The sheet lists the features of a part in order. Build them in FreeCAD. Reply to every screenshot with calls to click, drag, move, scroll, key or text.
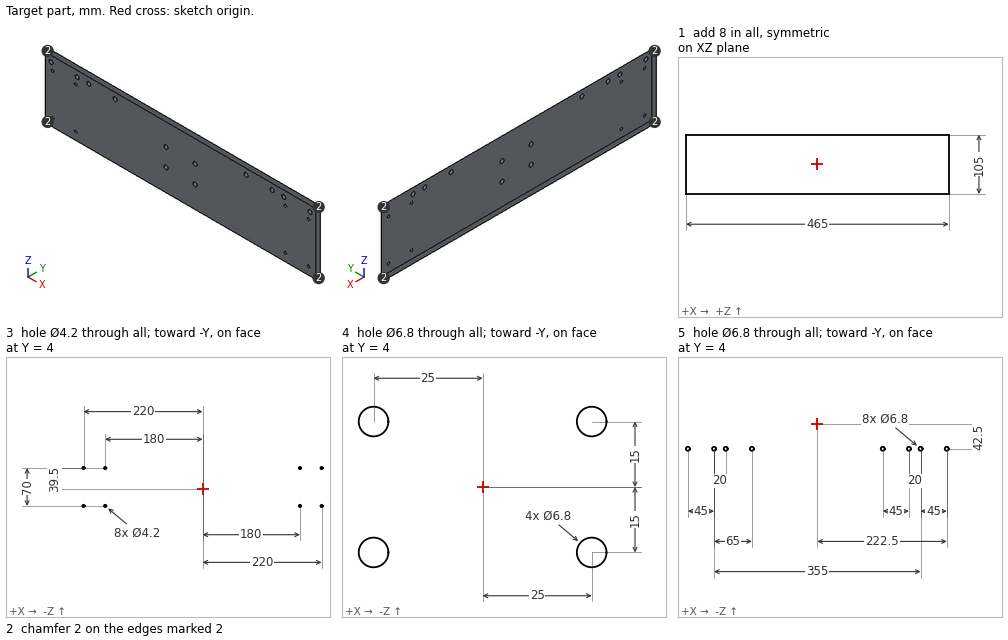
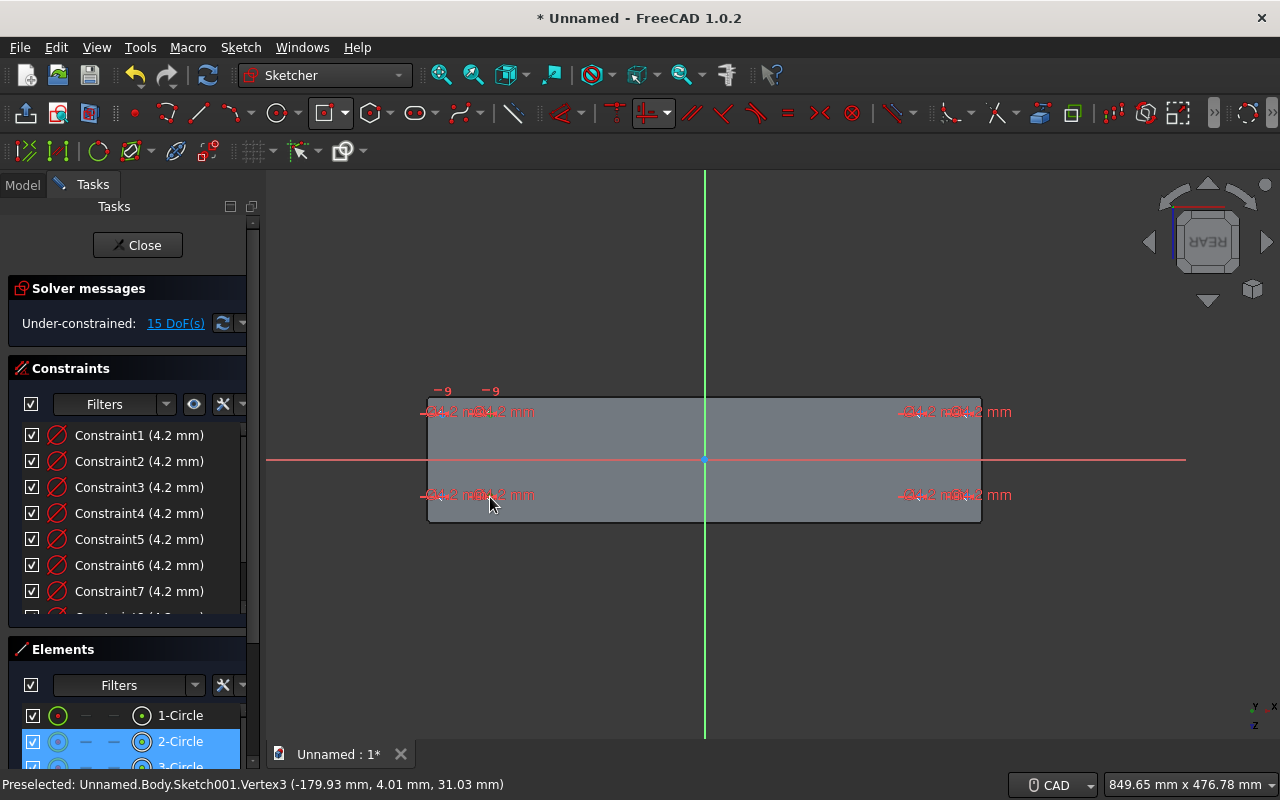
click(670, 114)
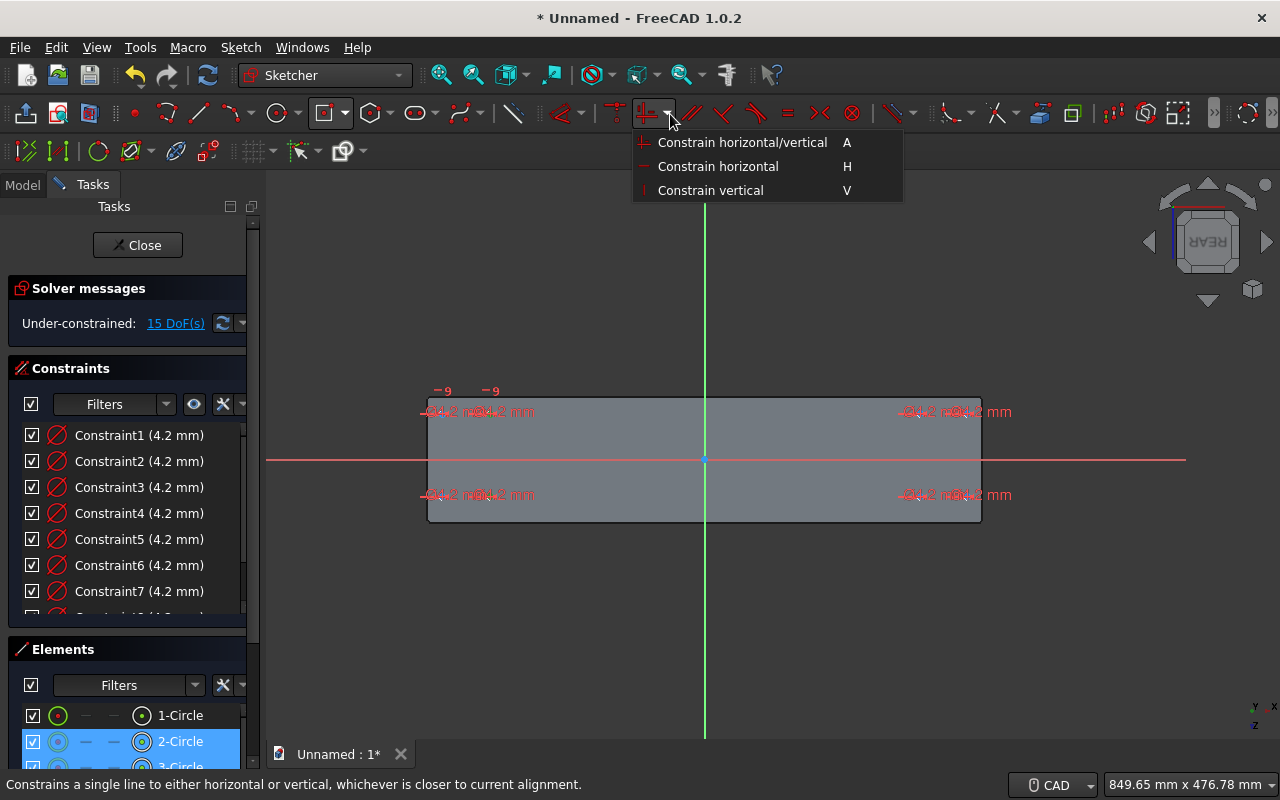
click(768, 190)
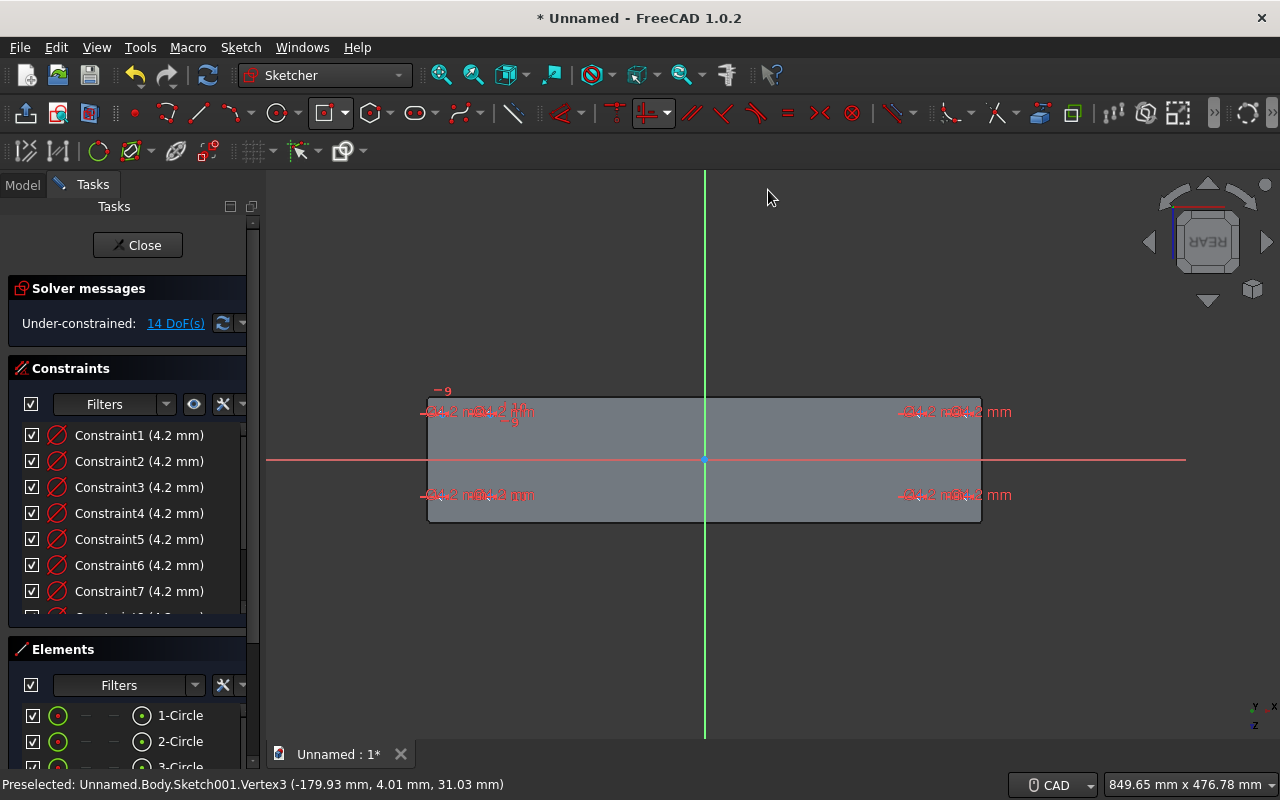
click(442, 414)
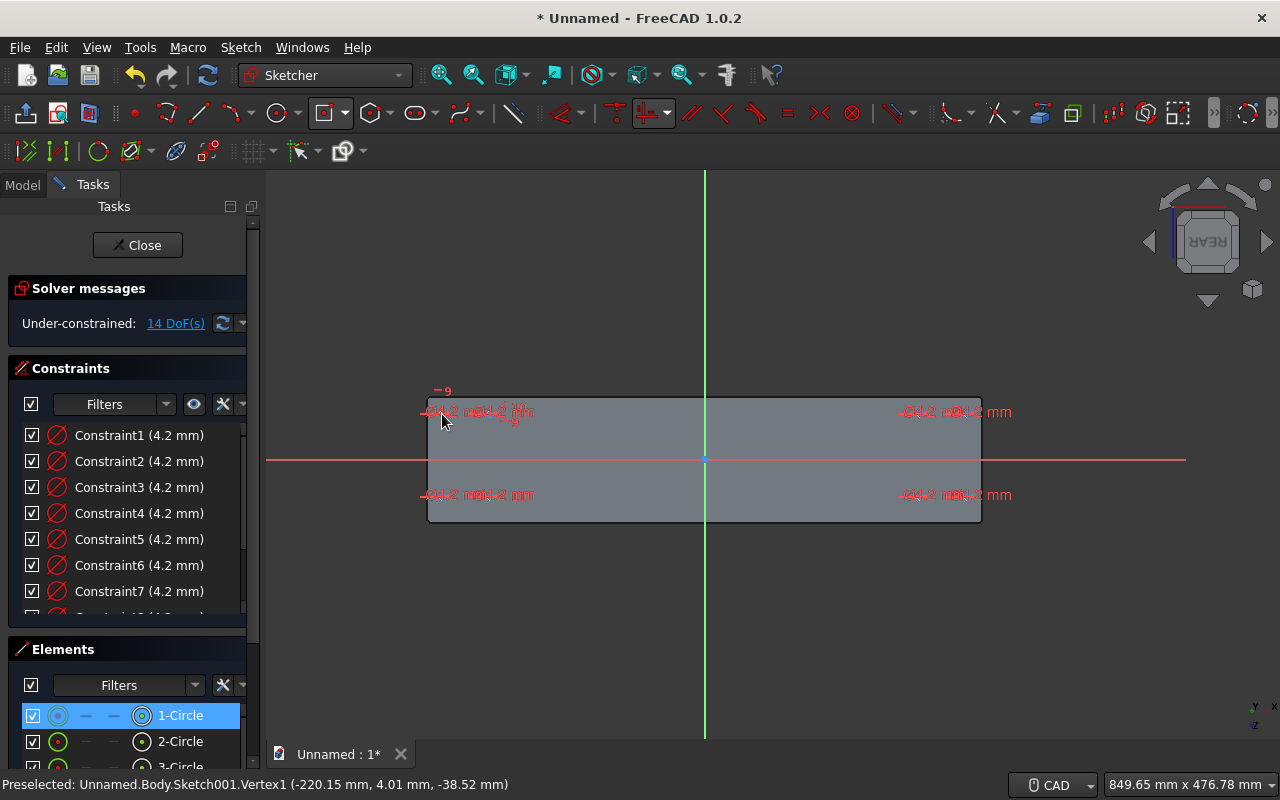
click(442, 497)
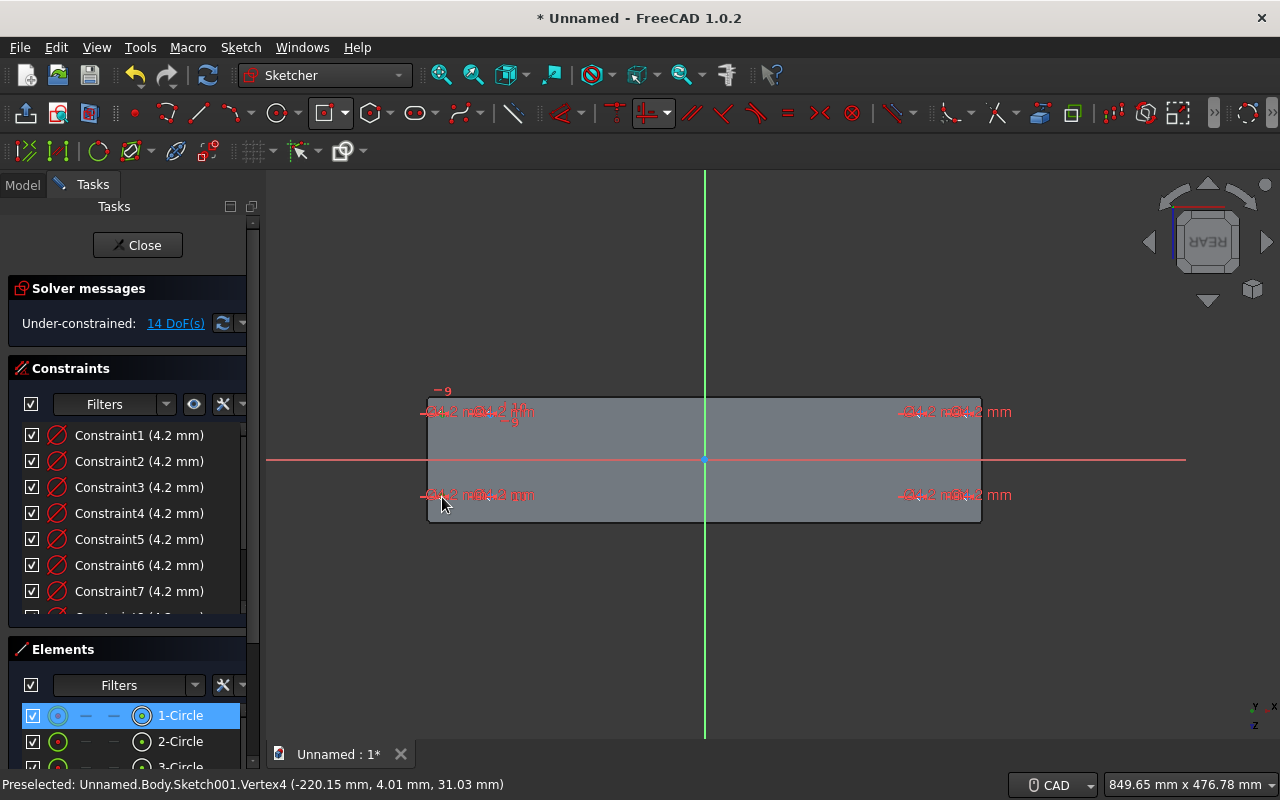
key(v)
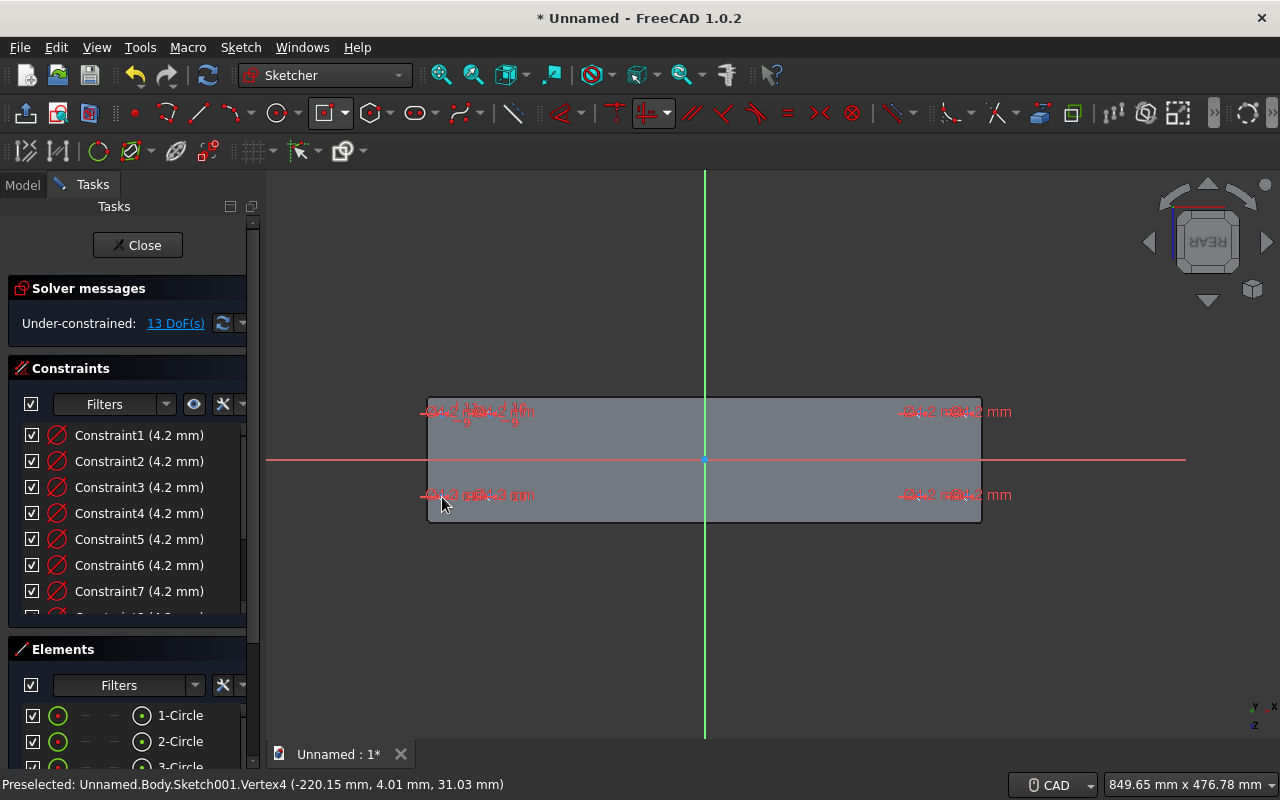
click(490, 497)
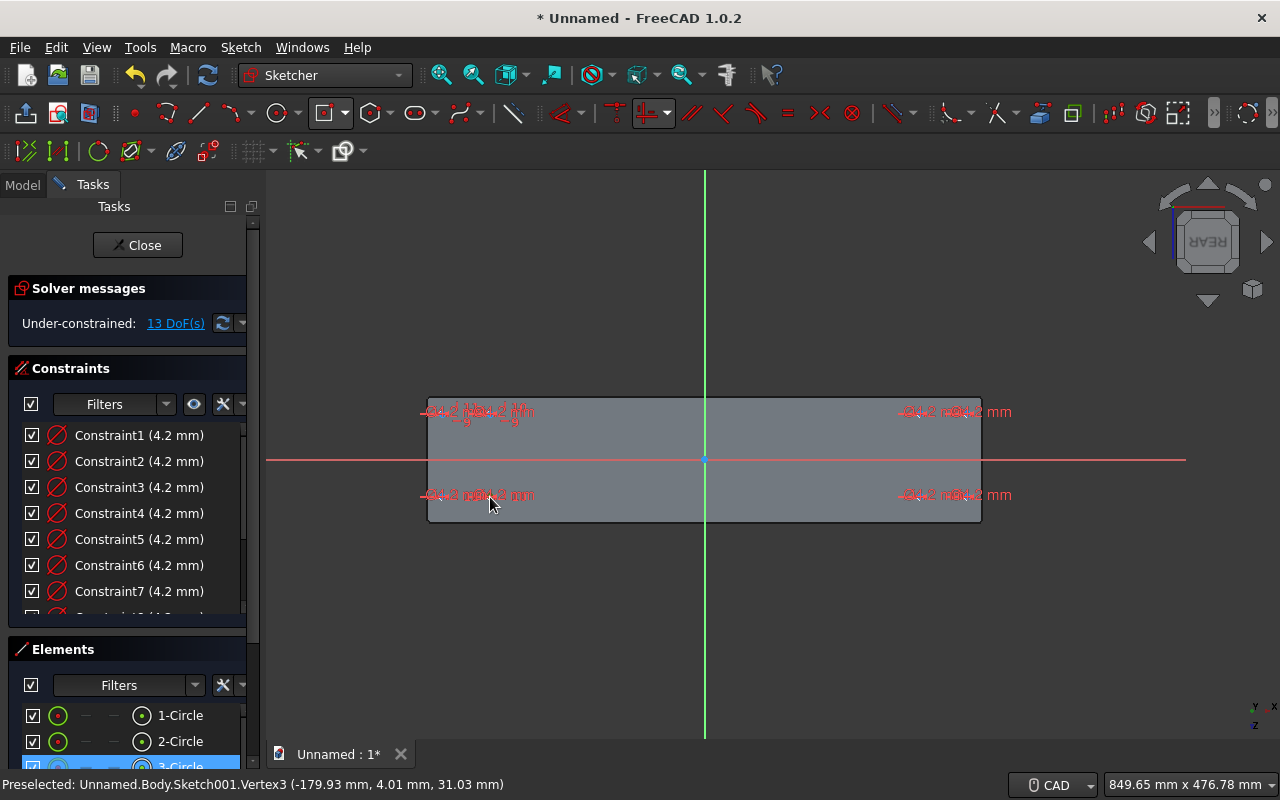
click(442, 497)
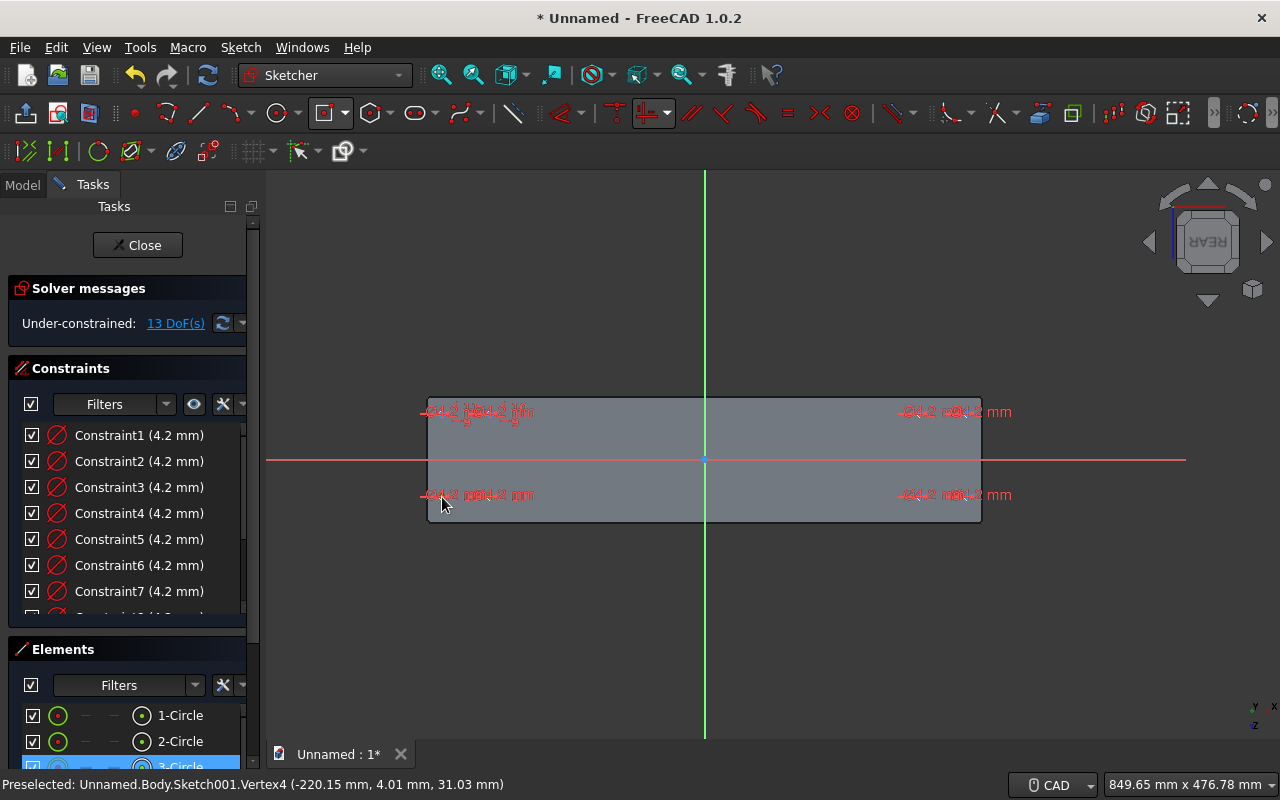
click(670, 114)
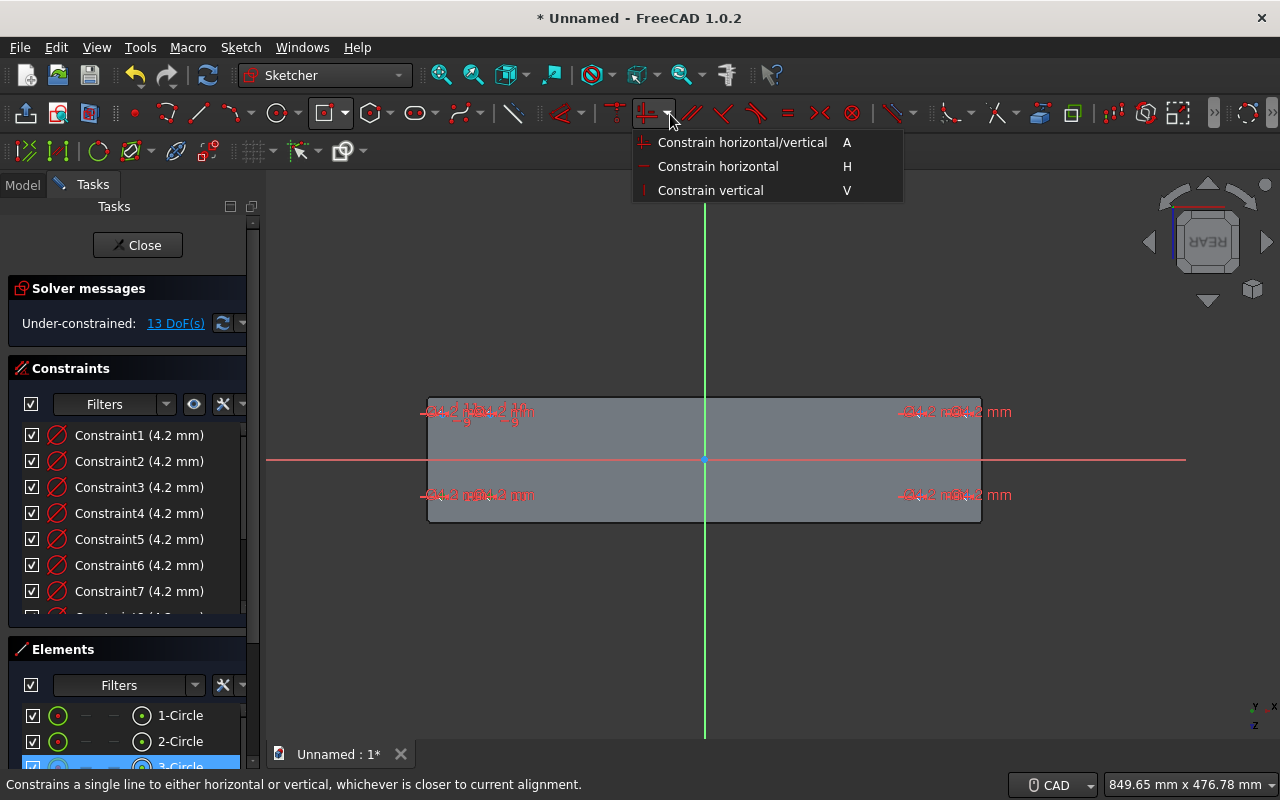
click(768, 166)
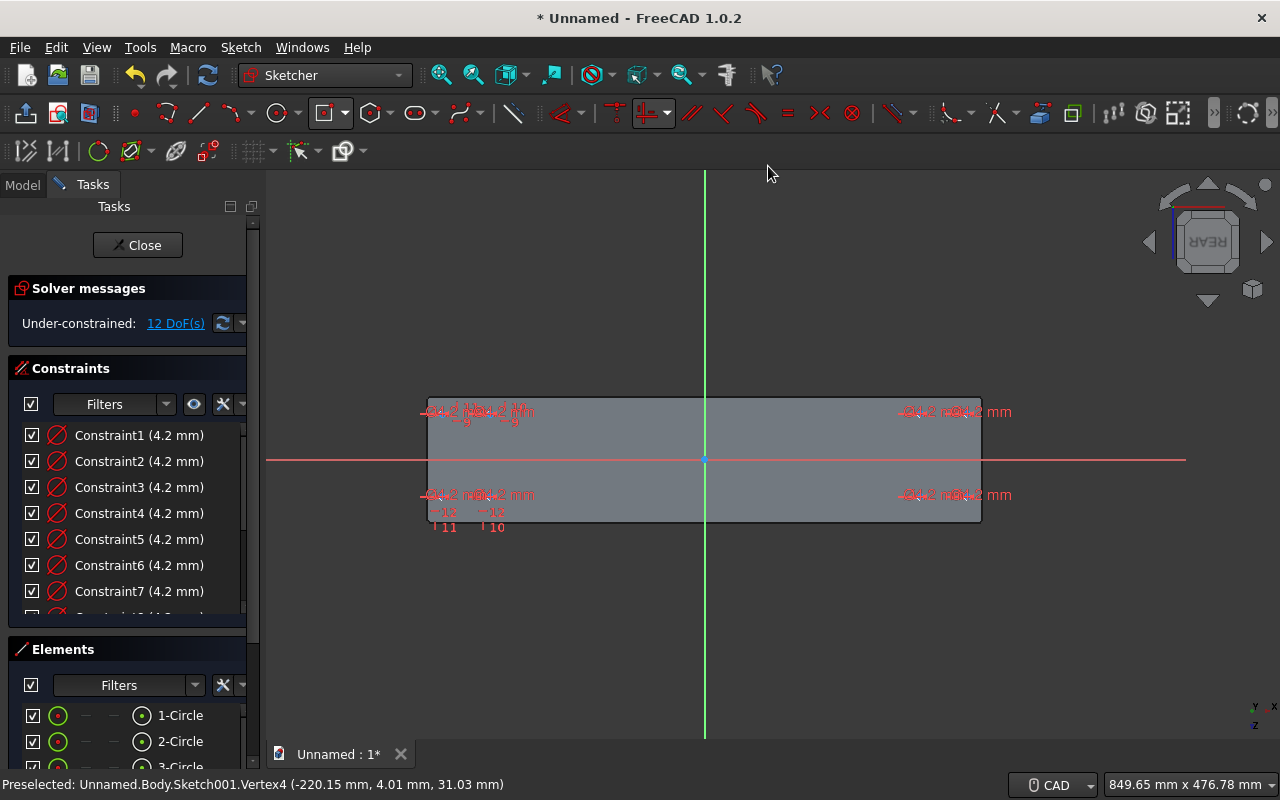
click(490, 497)